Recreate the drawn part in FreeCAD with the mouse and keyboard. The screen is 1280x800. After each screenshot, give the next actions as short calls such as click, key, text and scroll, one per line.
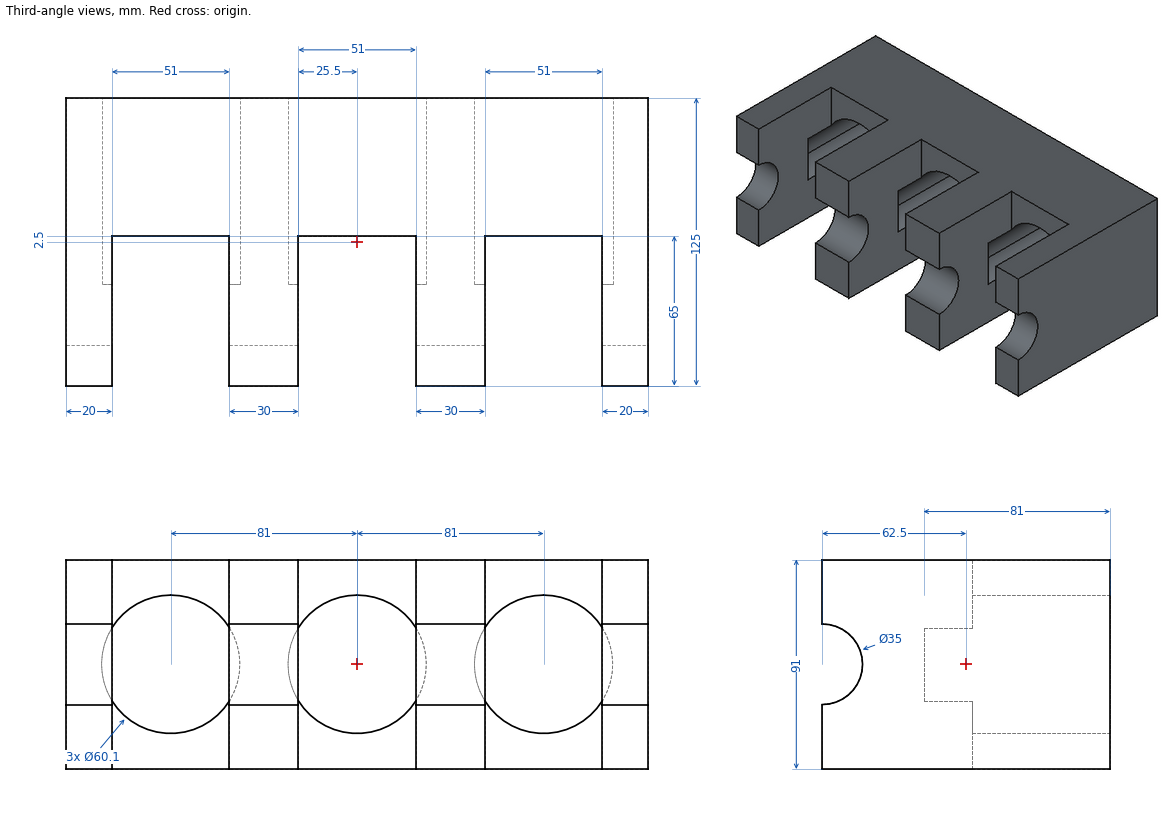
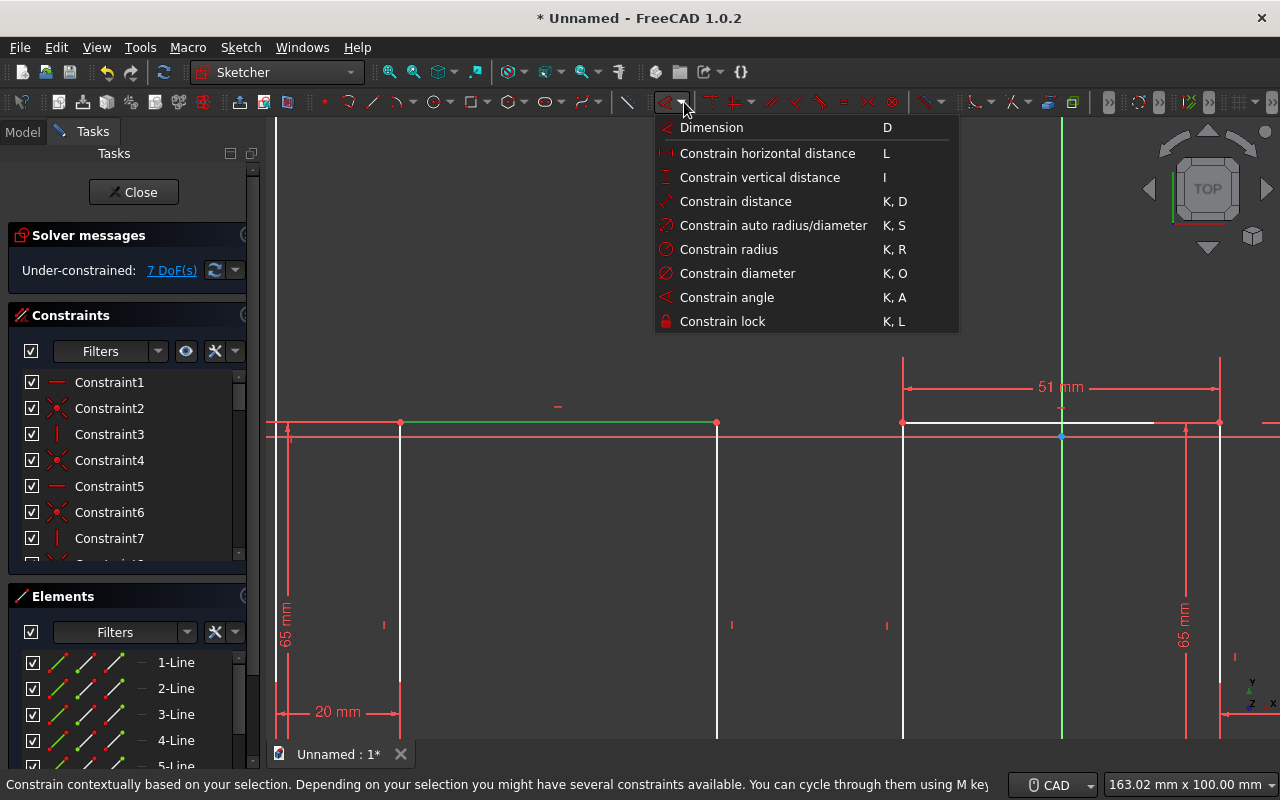
click(807, 153)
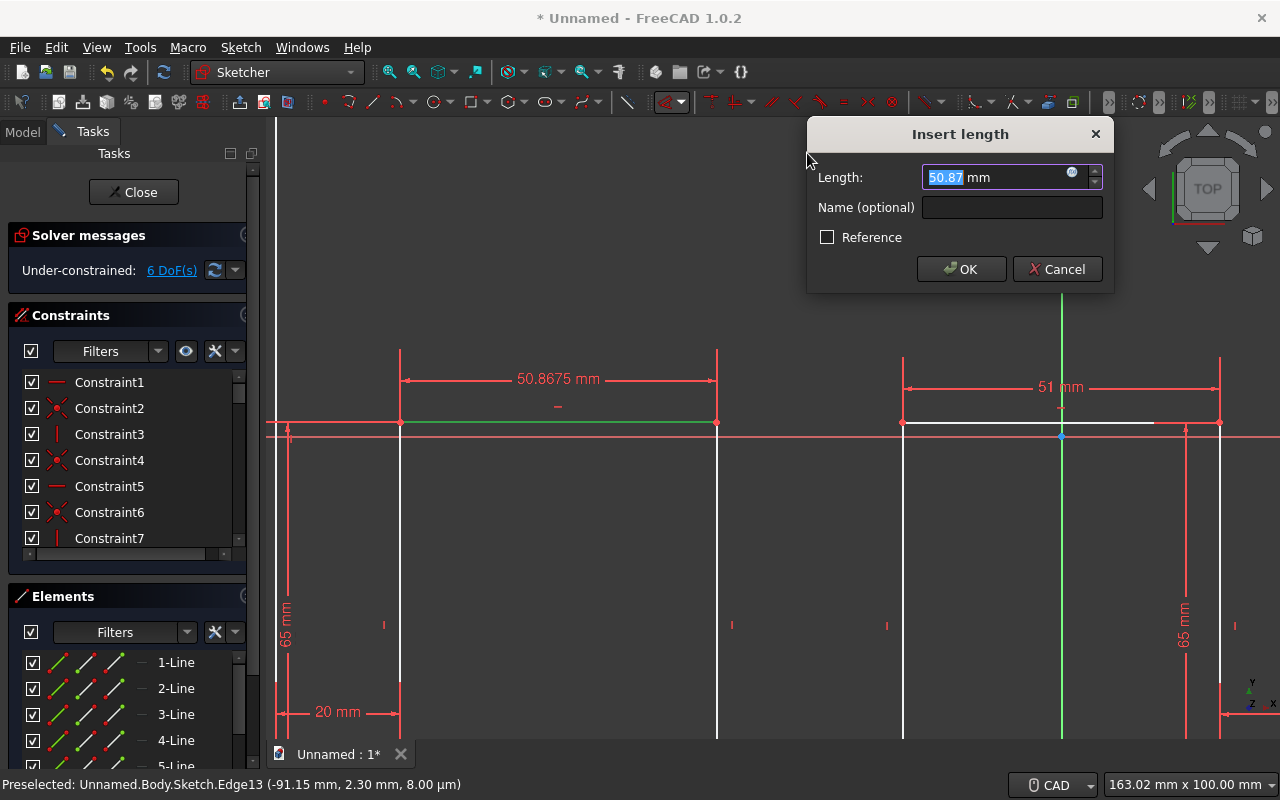
text(51)
key(Return)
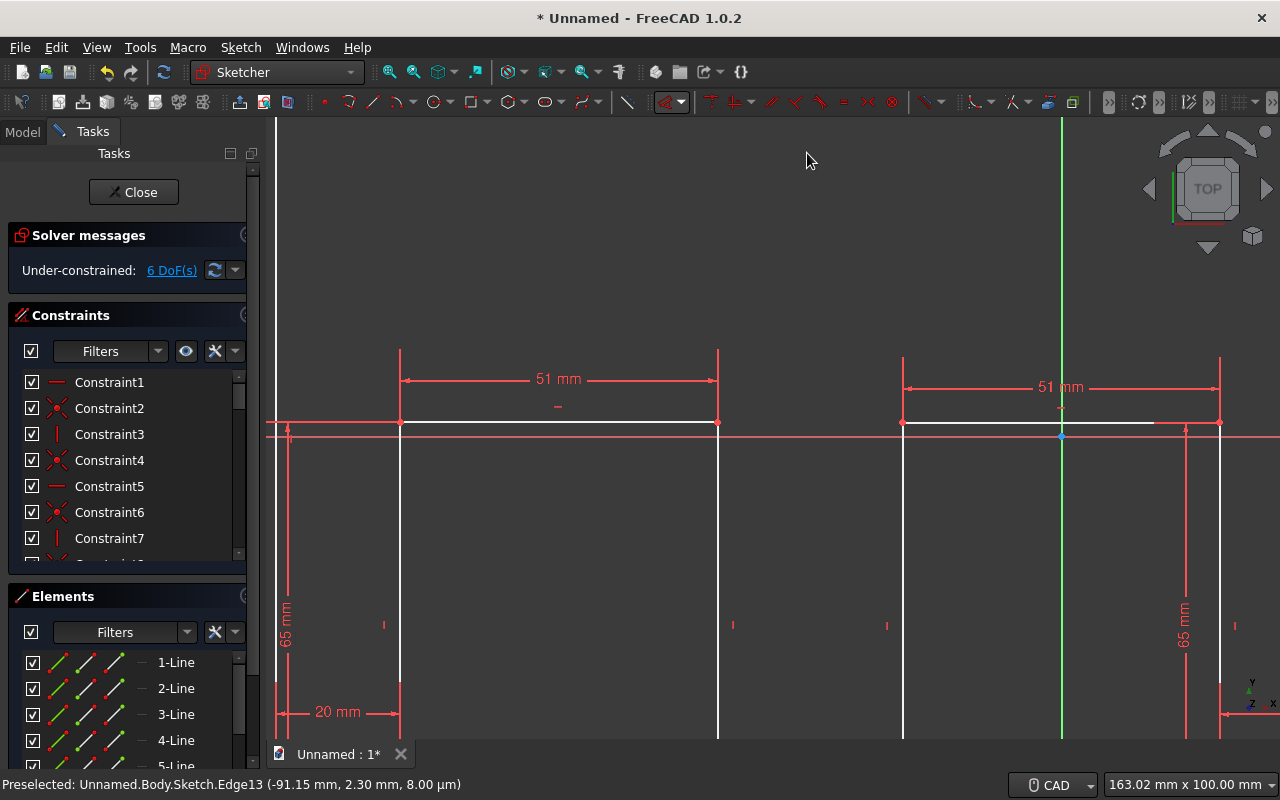
click(718, 544)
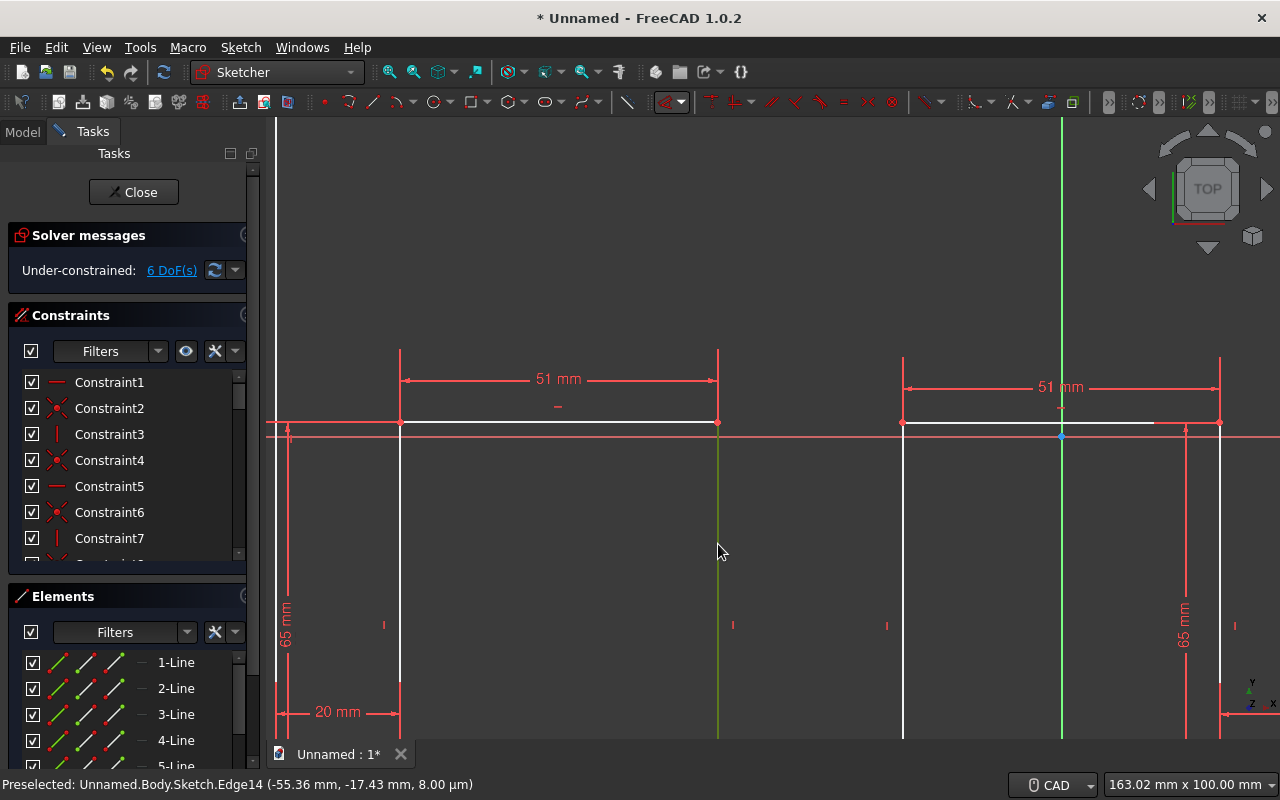
key(i)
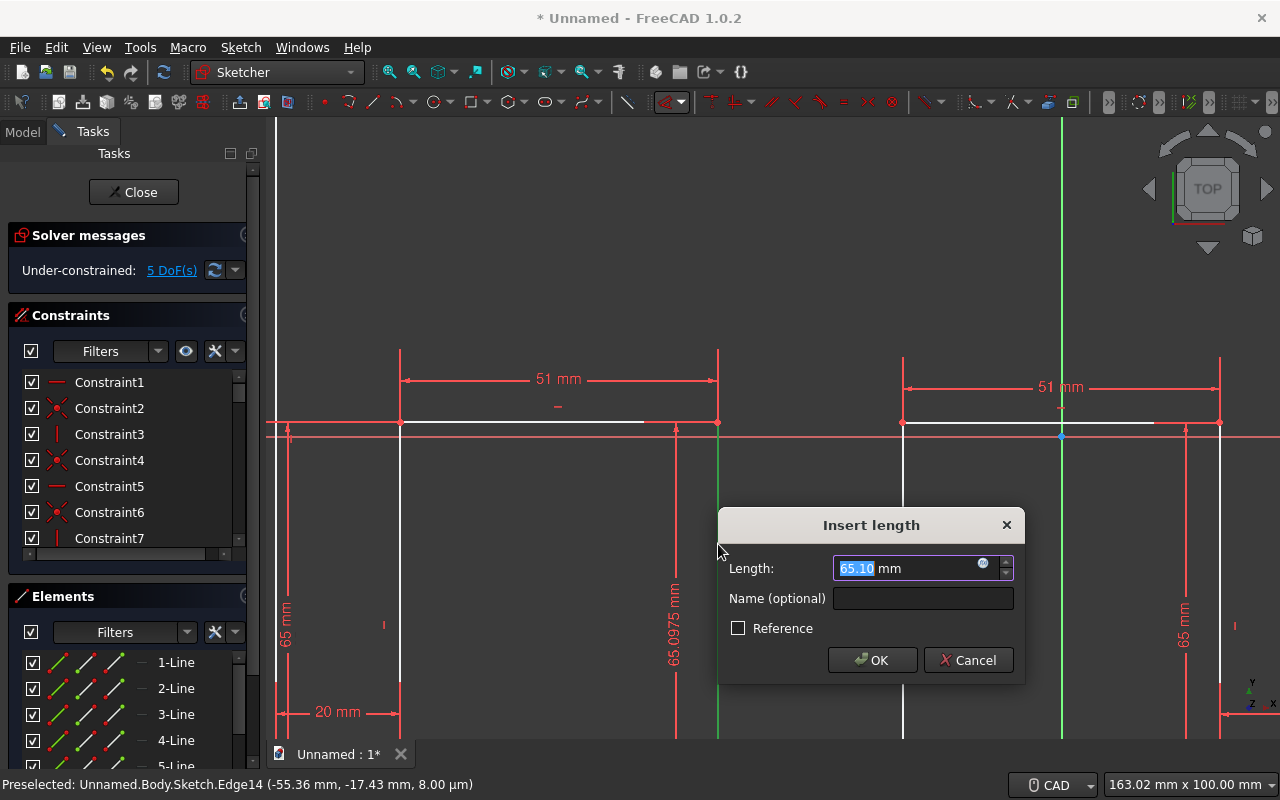
text(65)
key(Return)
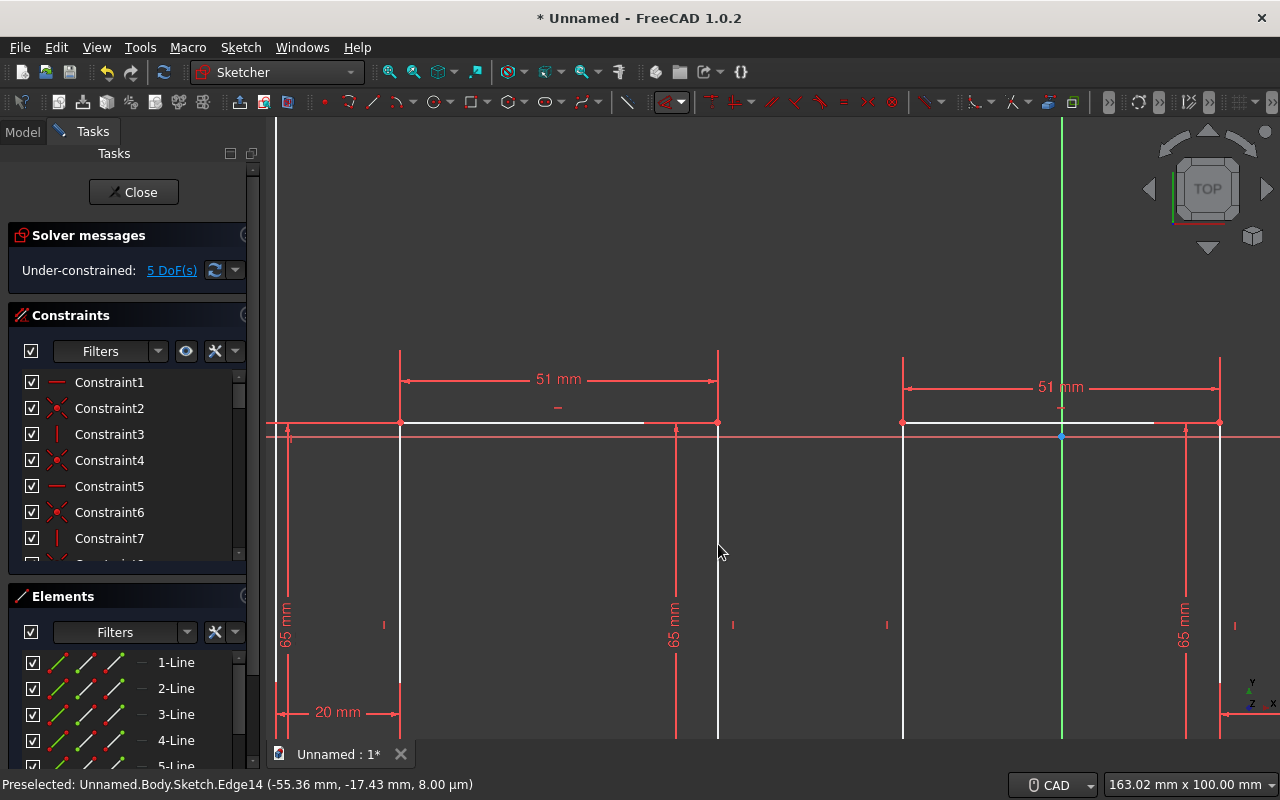
scroll(496, 423, down, 5)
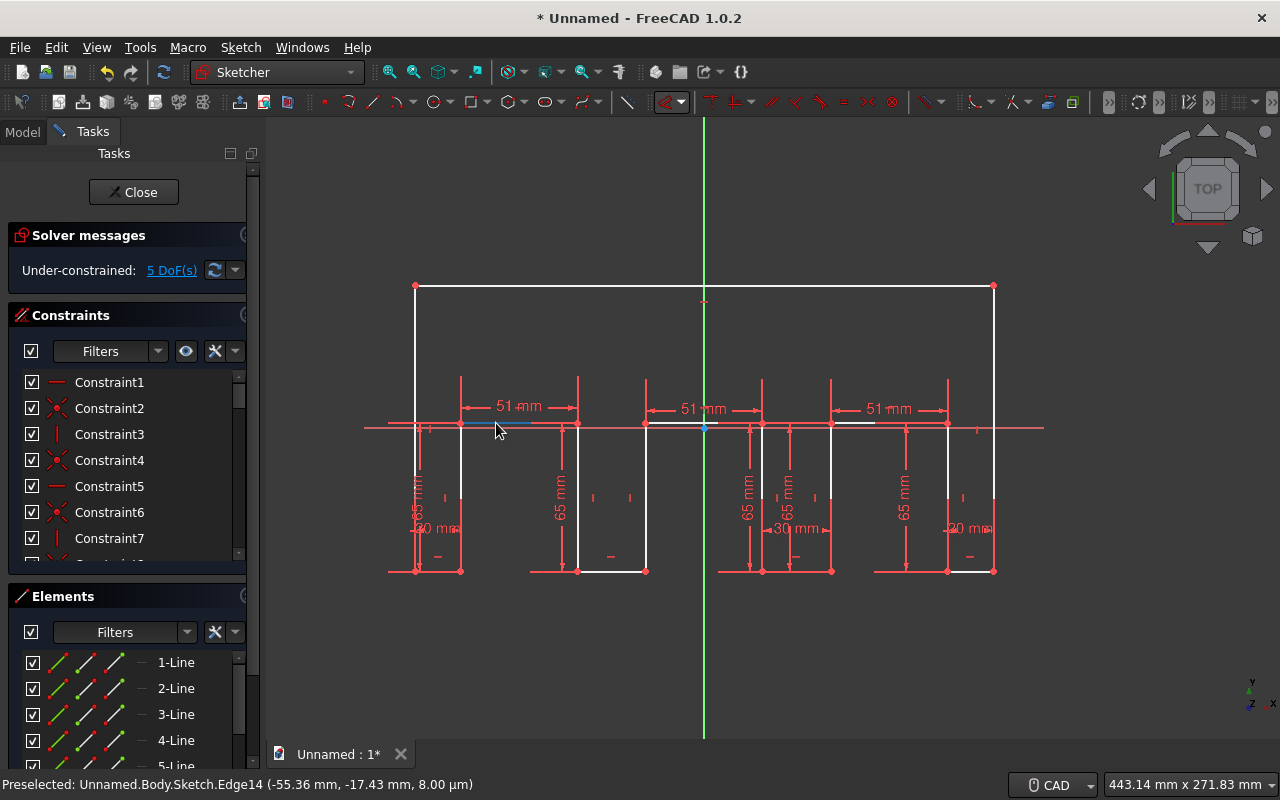
click(598, 572)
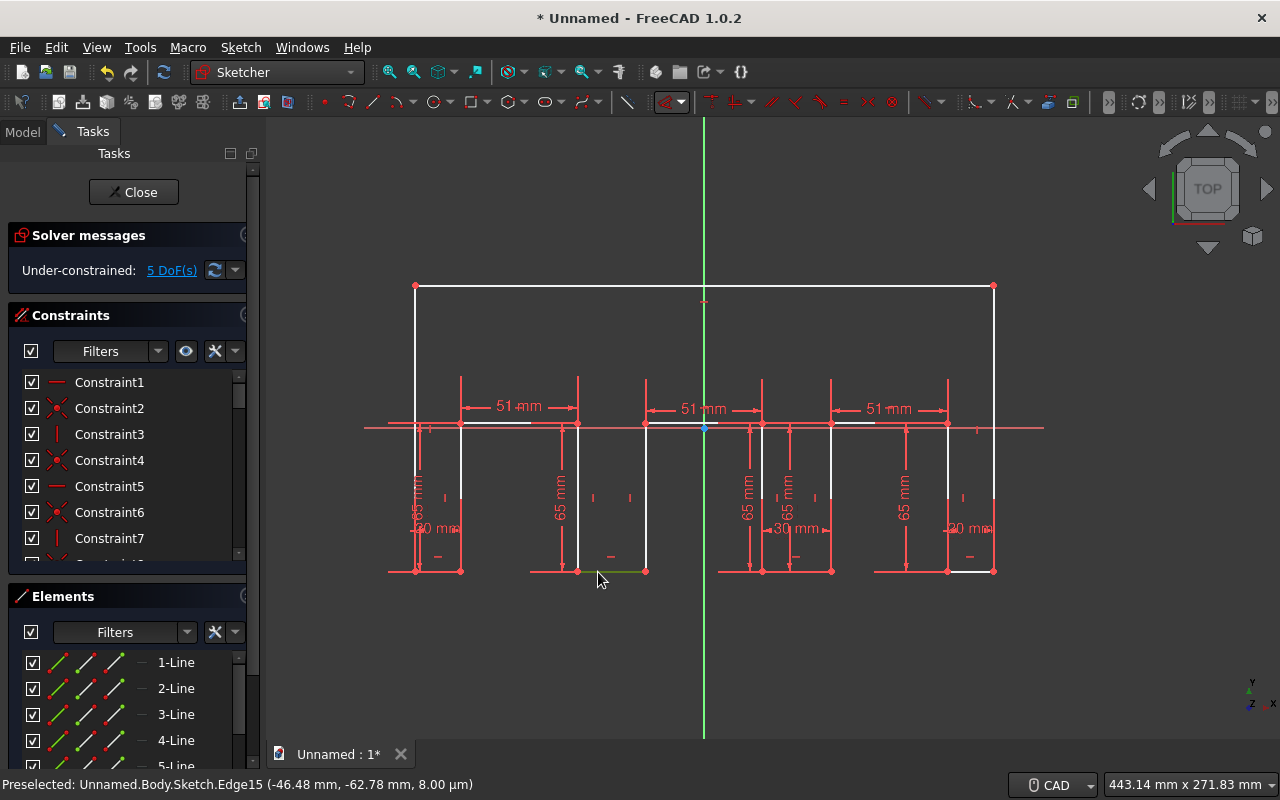
key(l)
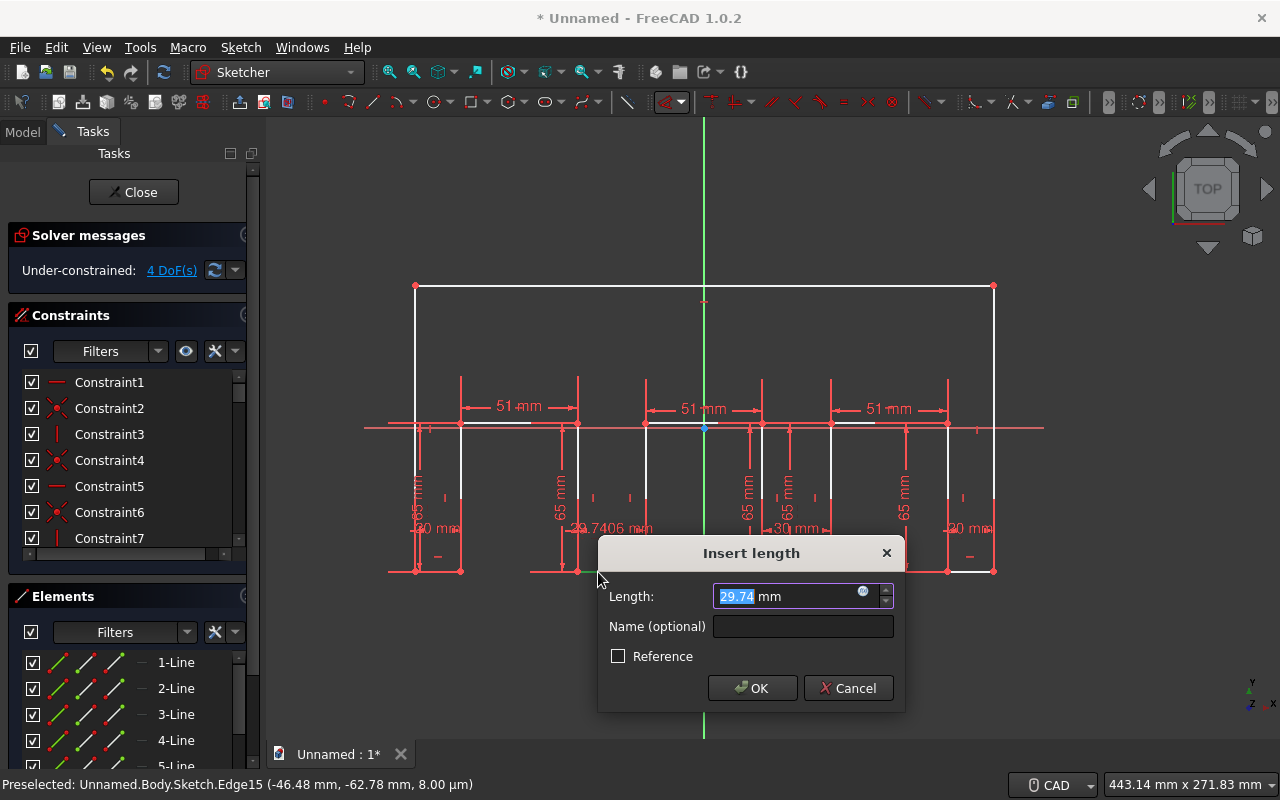
text(30)
key(Return)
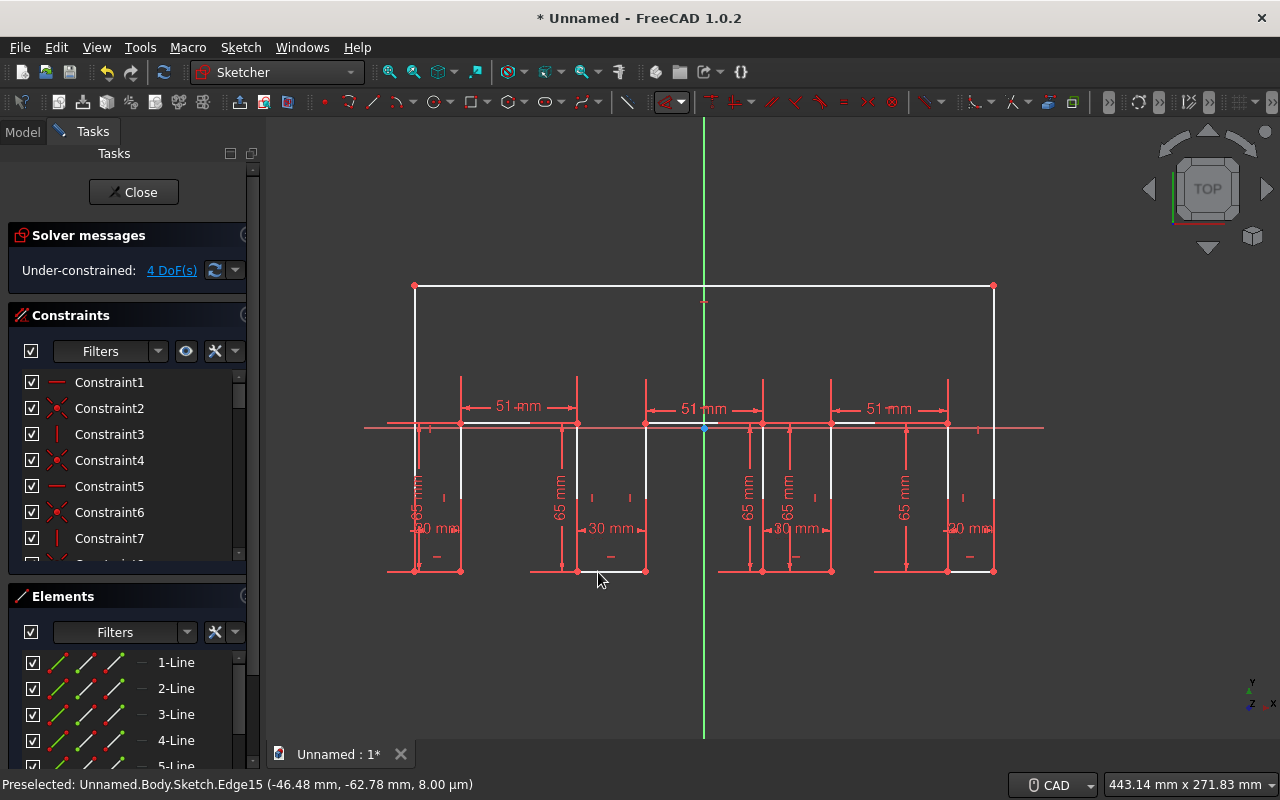
click(646, 527)